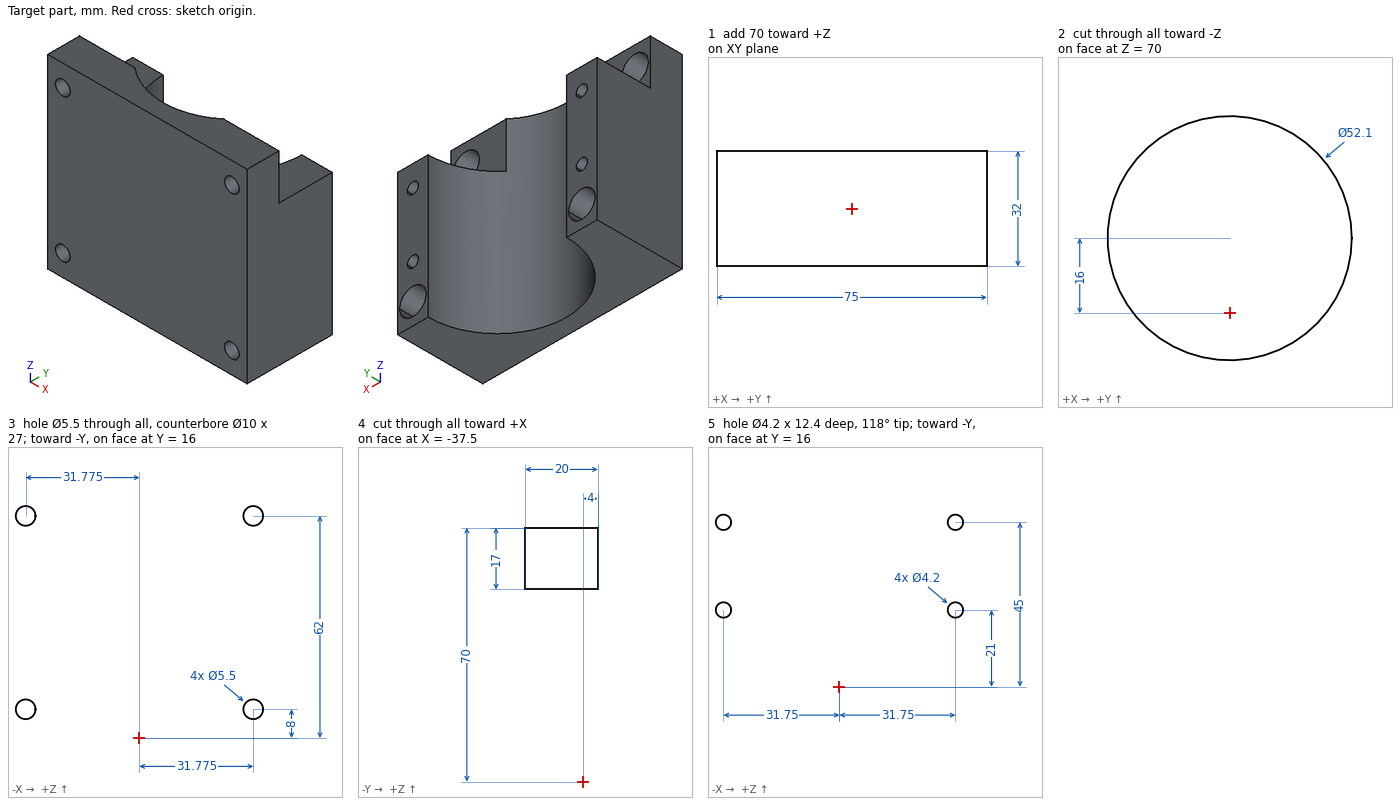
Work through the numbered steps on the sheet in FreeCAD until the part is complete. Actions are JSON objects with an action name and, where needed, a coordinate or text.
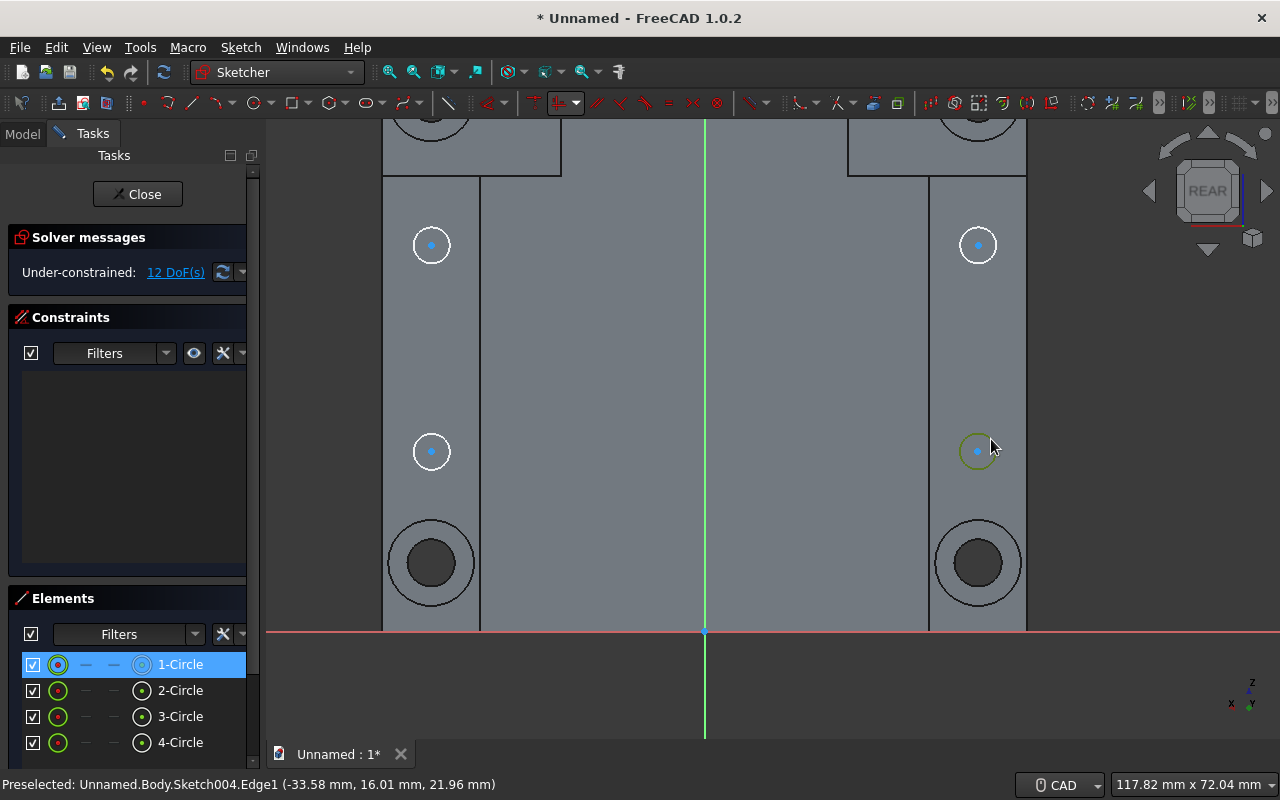
{"action": "left_click", "coordinate": [991, 233]}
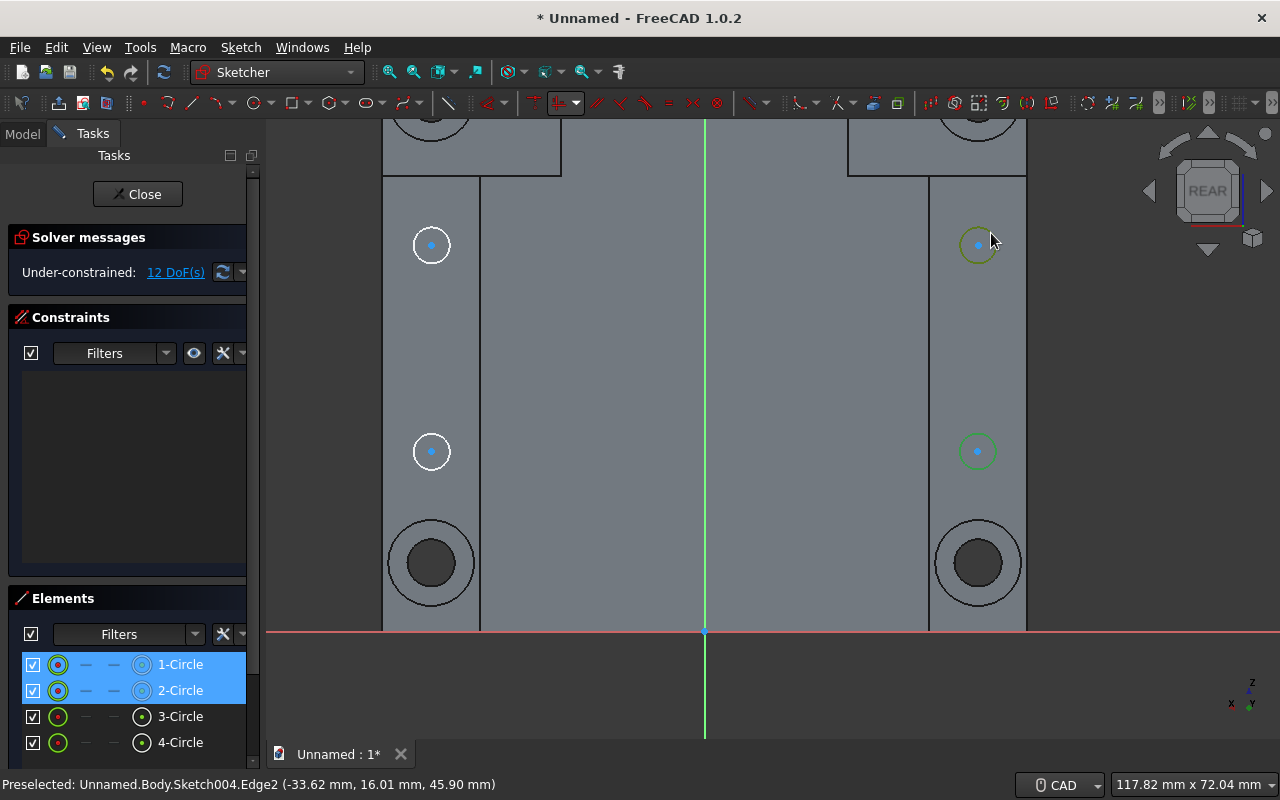
{"action": "left_click", "coordinate": [444, 439]}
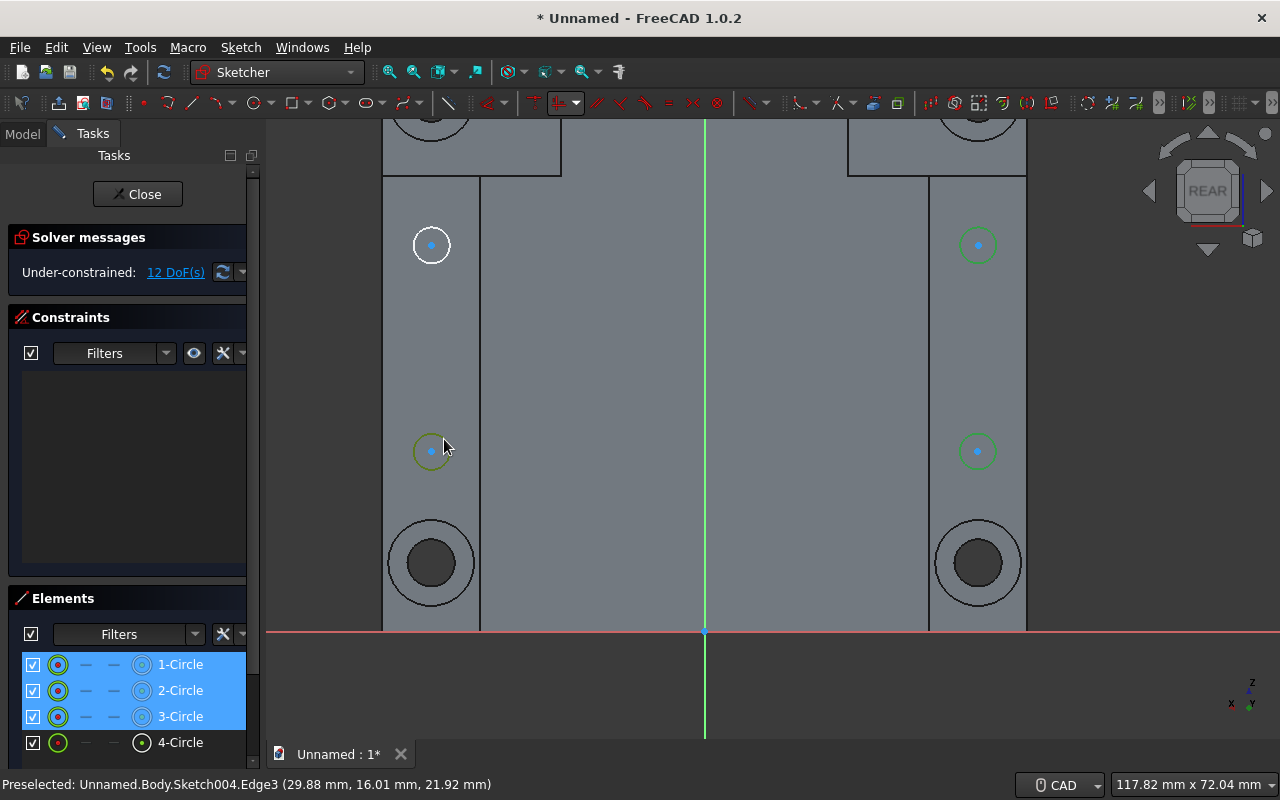
{"action": "left_click", "coordinate": [444, 233]}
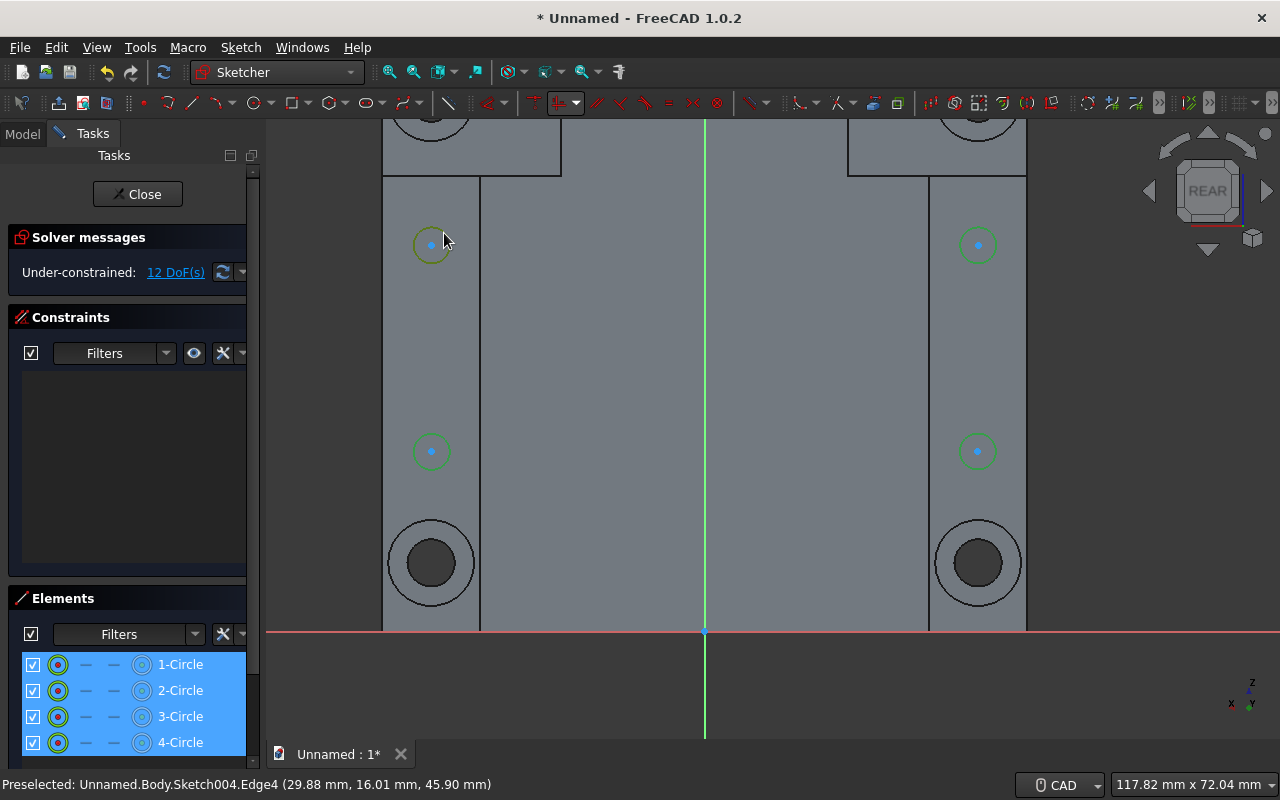
{"action": "left_click", "coordinate": [670, 104]}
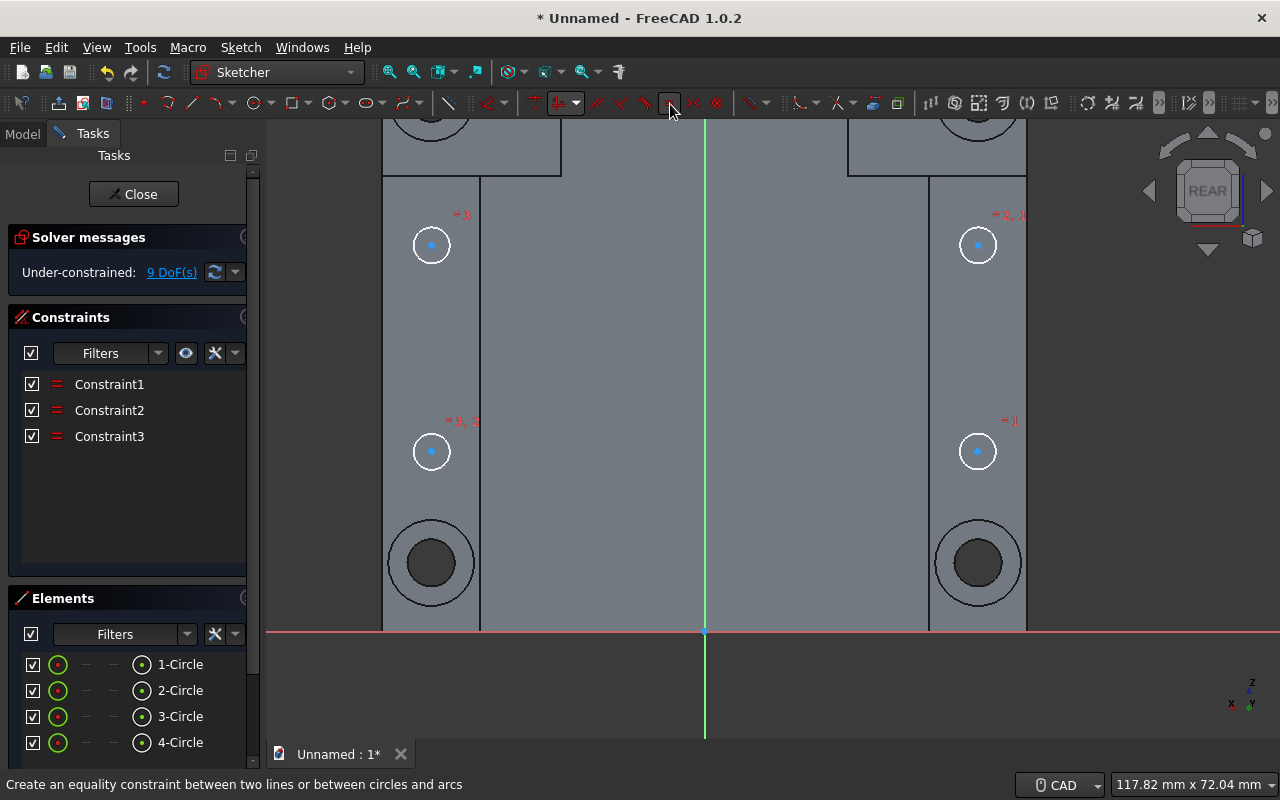
{"action": "left_click", "coordinate": [978, 452]}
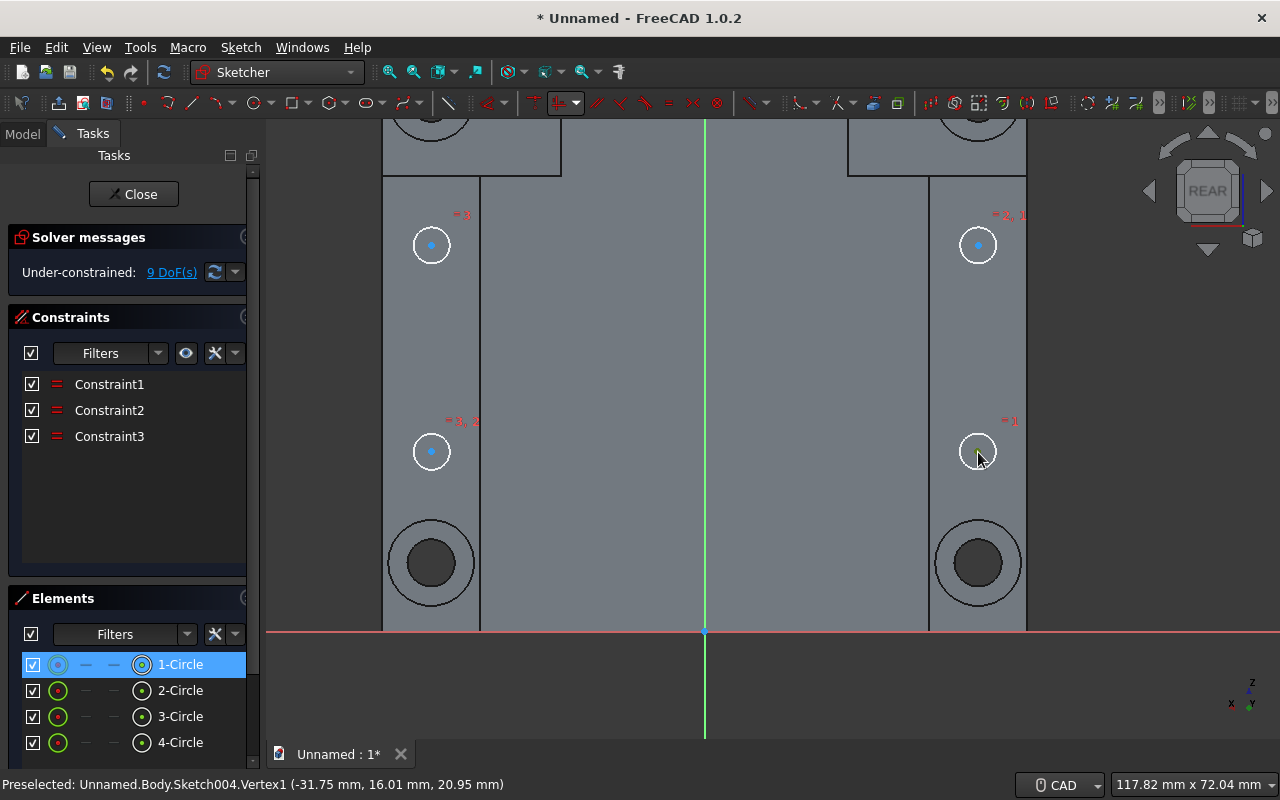
{"action": "left_click", "coordinate": [978, 245]}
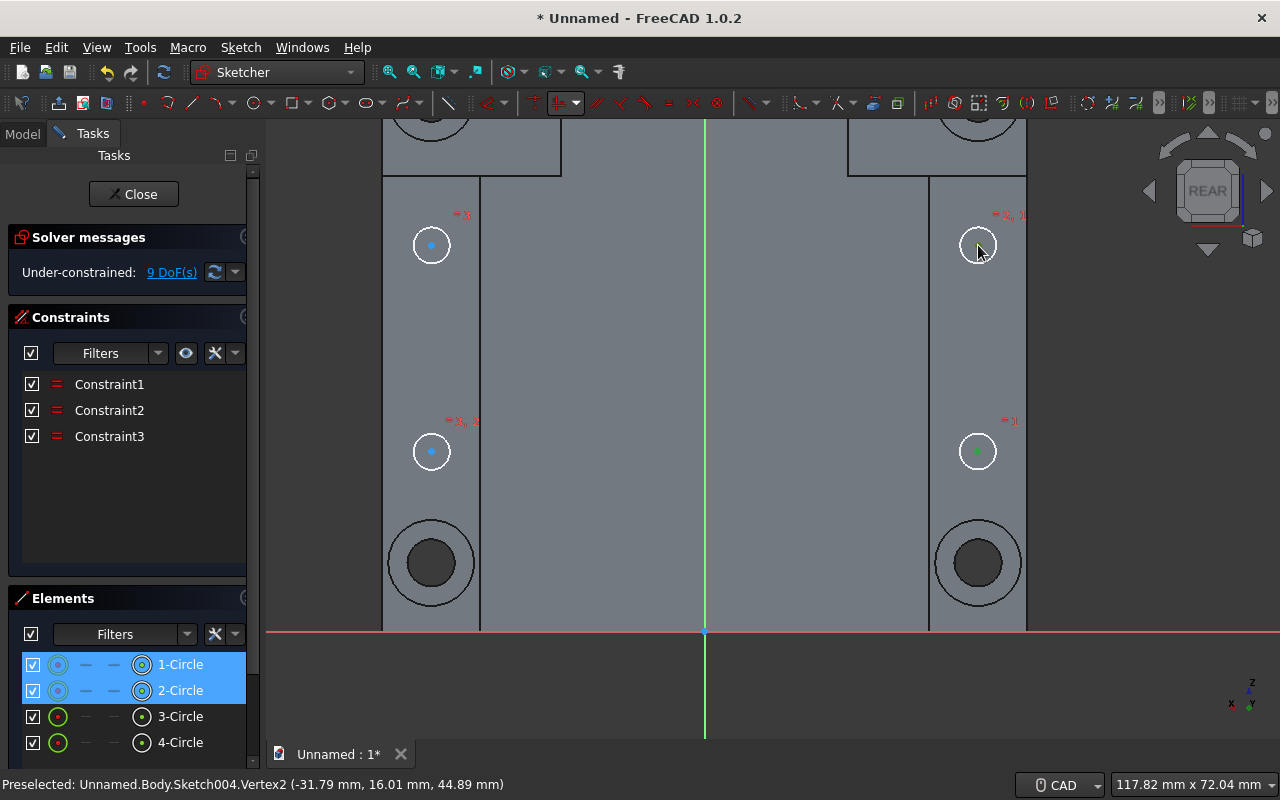
{"action": "left_click", "coordinate": [578, 104]}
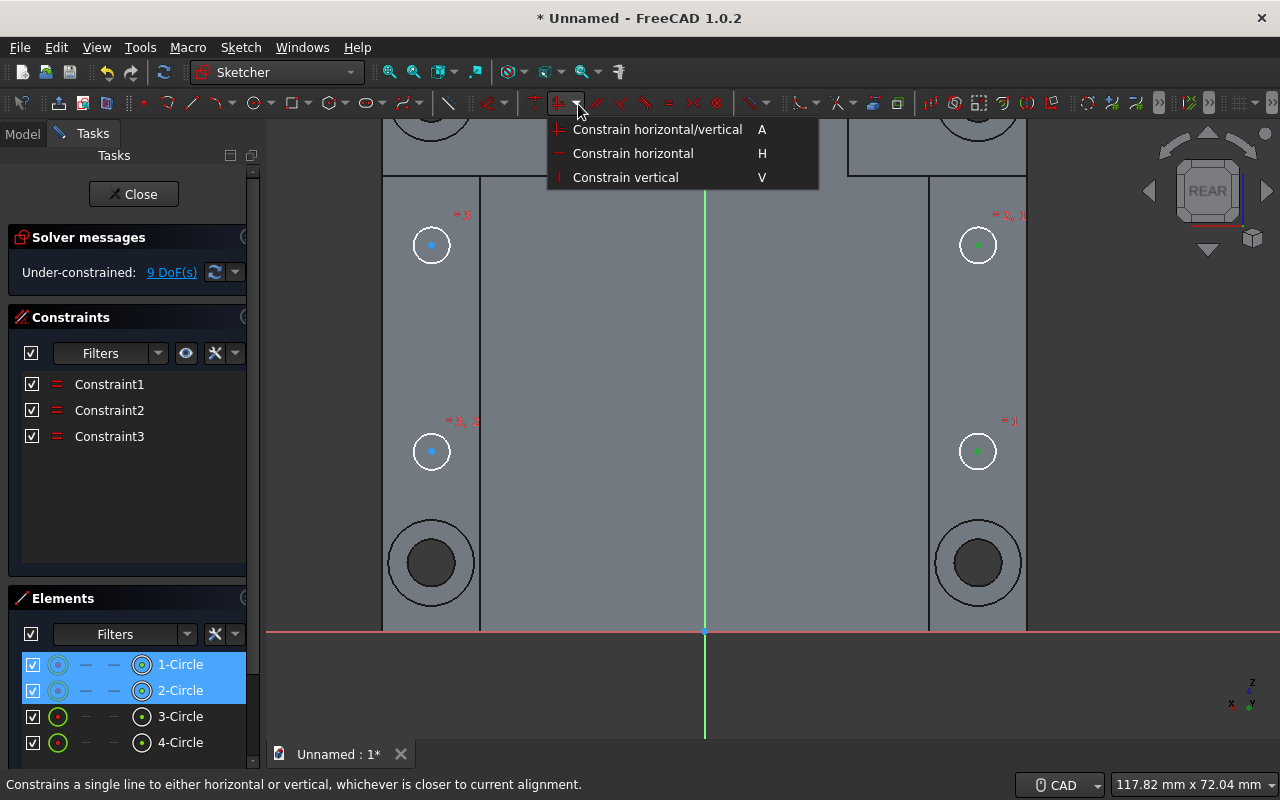
{"action": "left_click", "coordinate": [683, 177]}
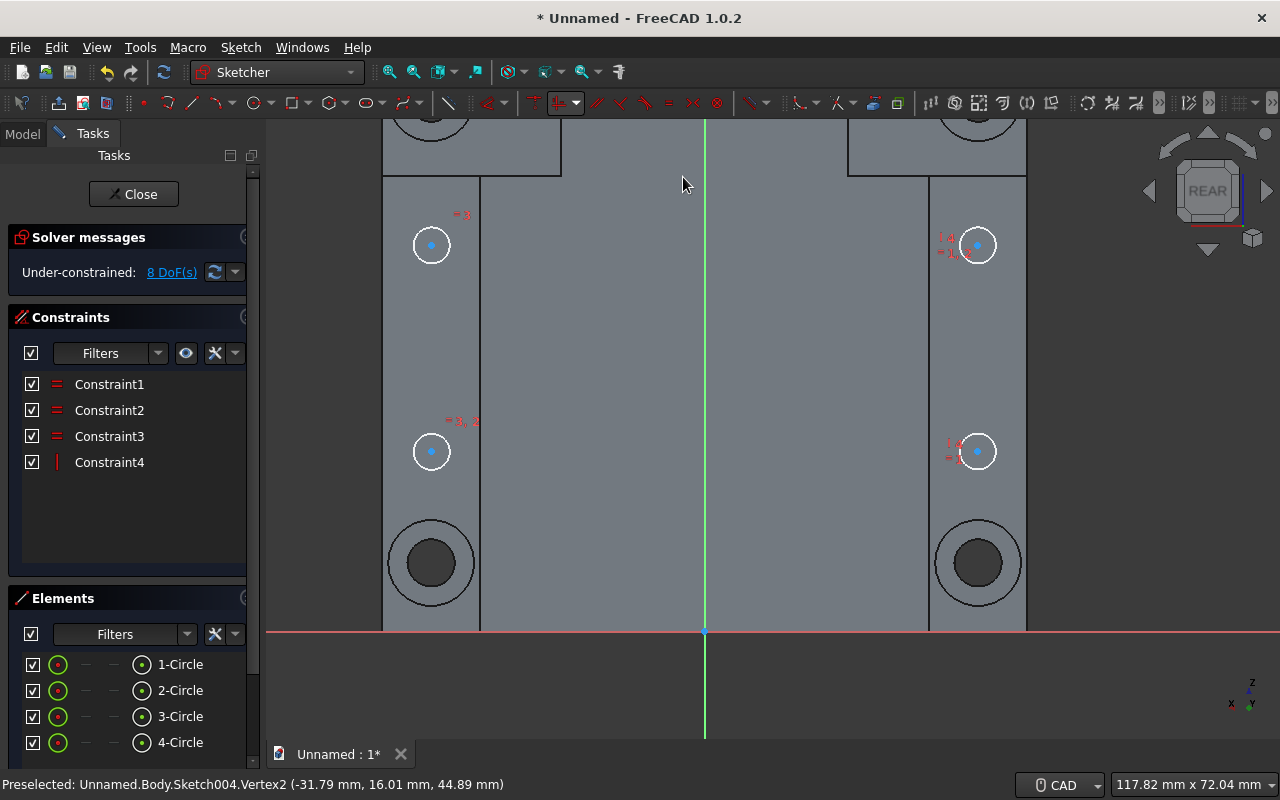
{"action": "left_click", "coordinate": [978, 452]}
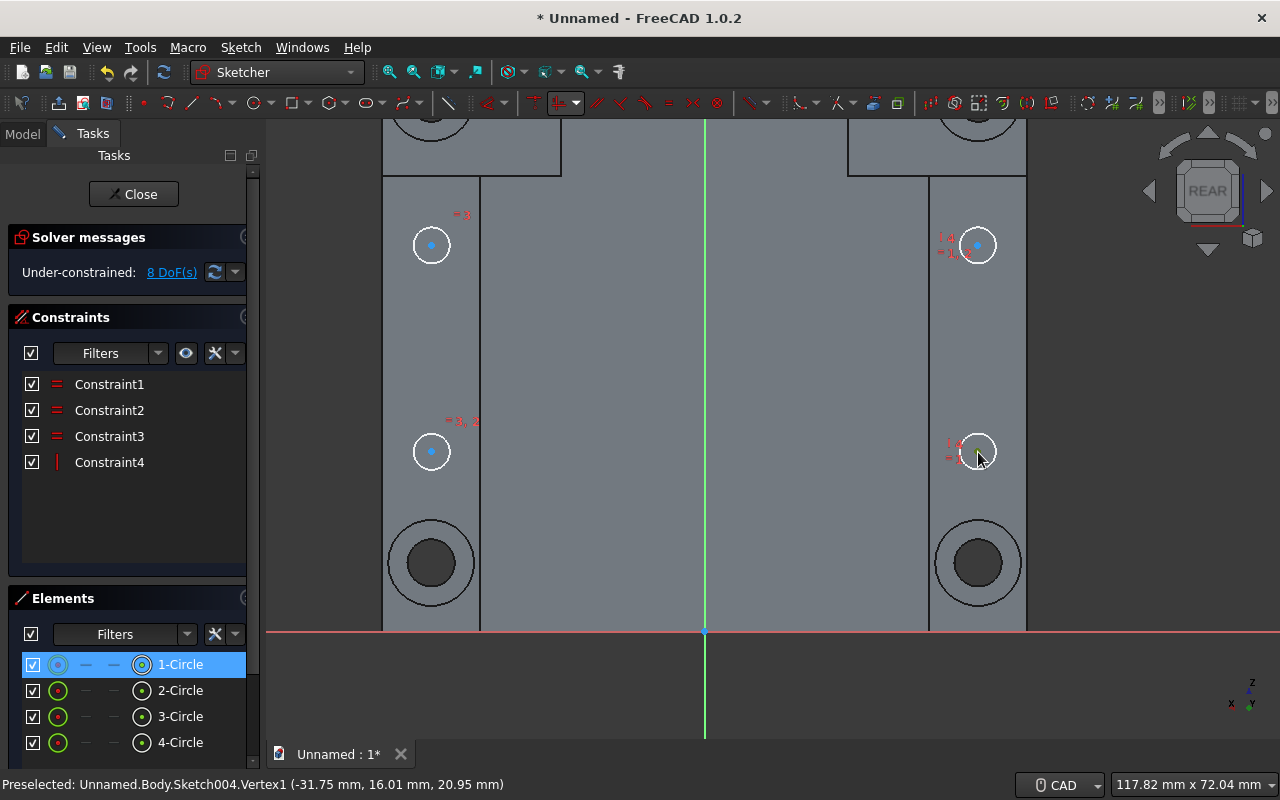
{"action": "left_click", "coordinate": [432, 452]}